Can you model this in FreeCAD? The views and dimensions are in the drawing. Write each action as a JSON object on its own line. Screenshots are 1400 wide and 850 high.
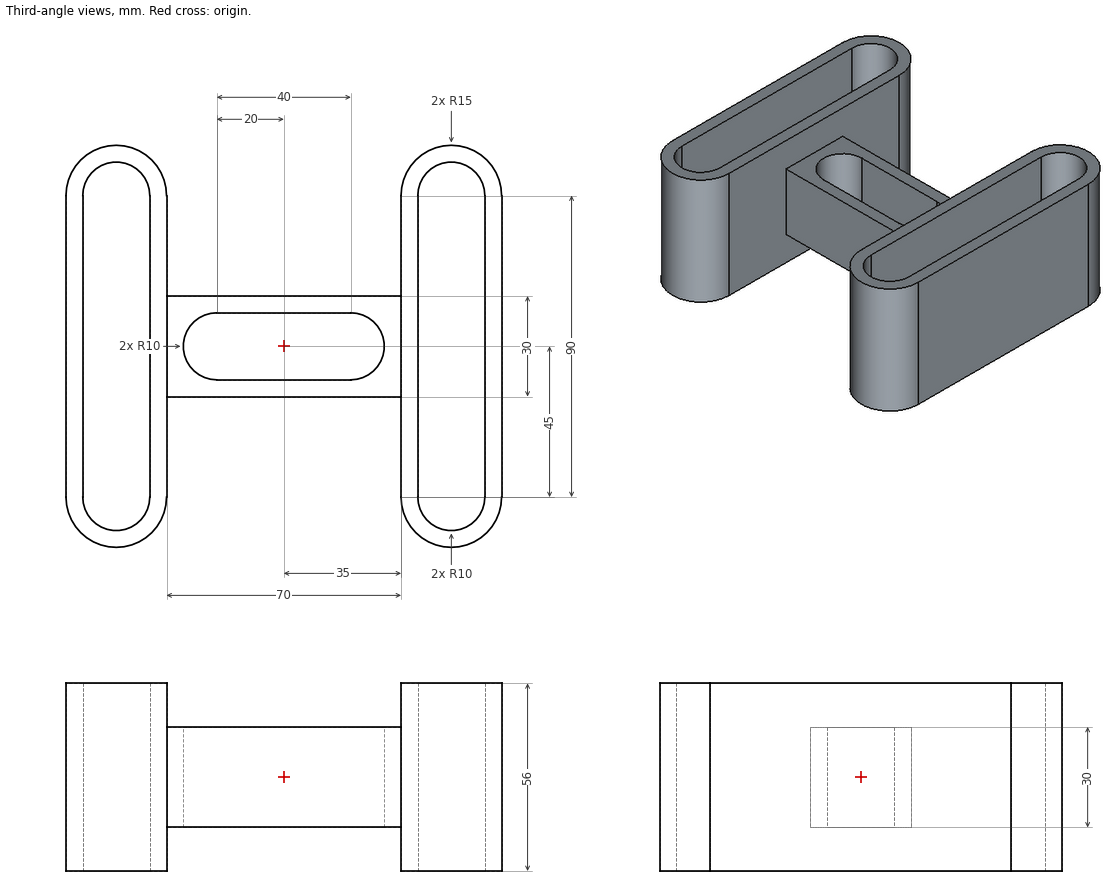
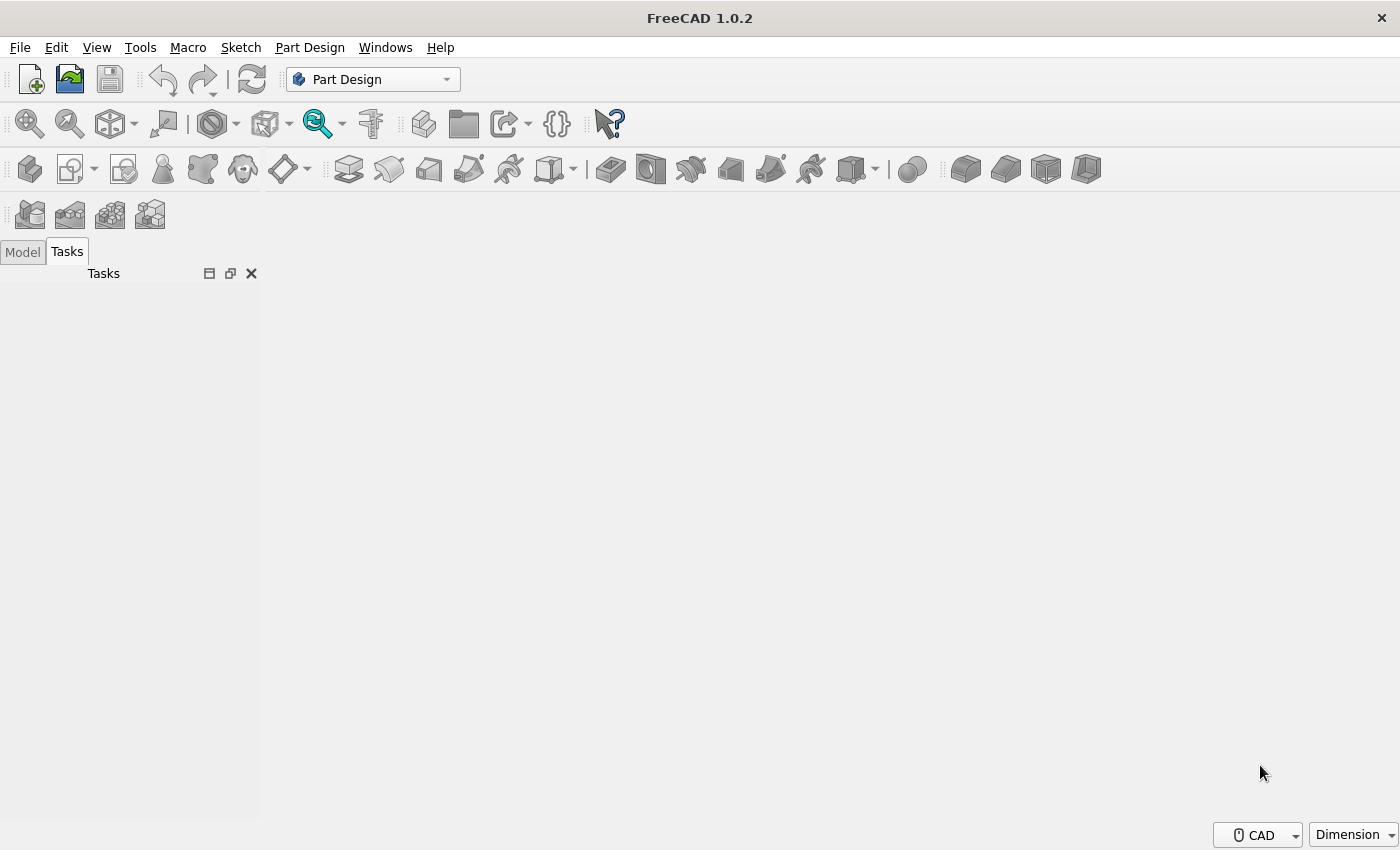
{"action": "left_click", "coordinate": [30, 80]}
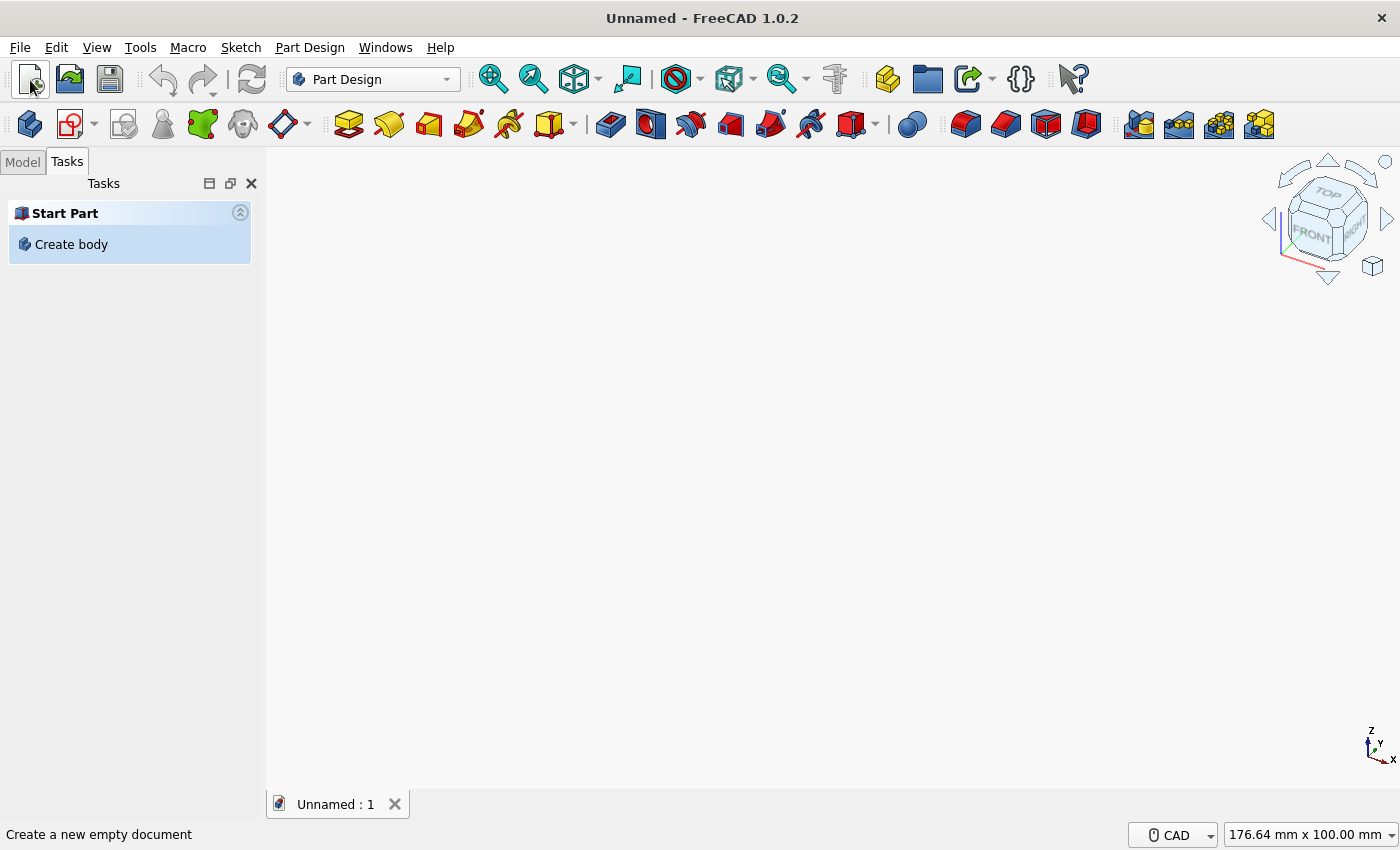
{"action": "left_click", "coordinate": [70, 124]}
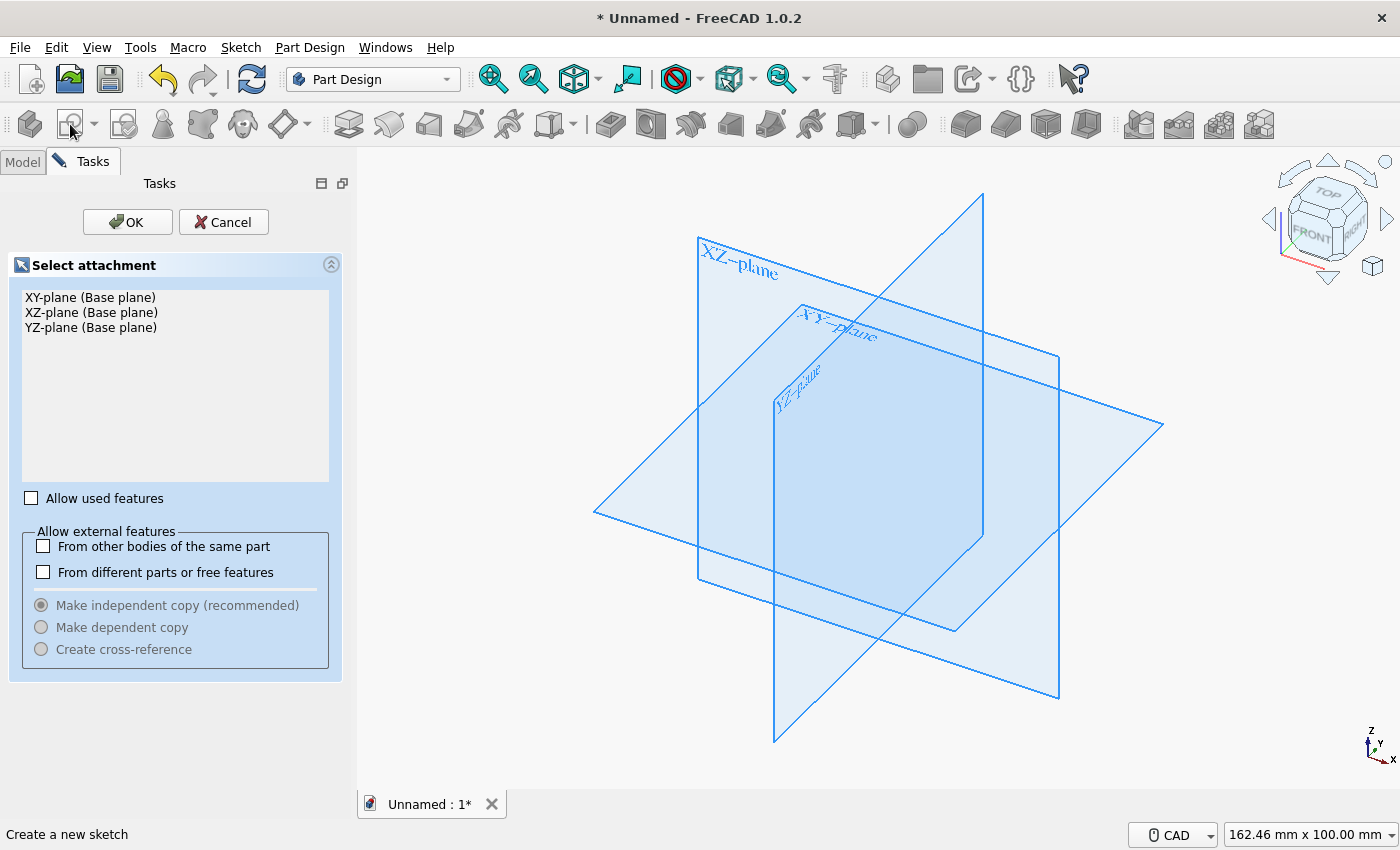
{"action": "left_click", "coordinate": [82, 298]}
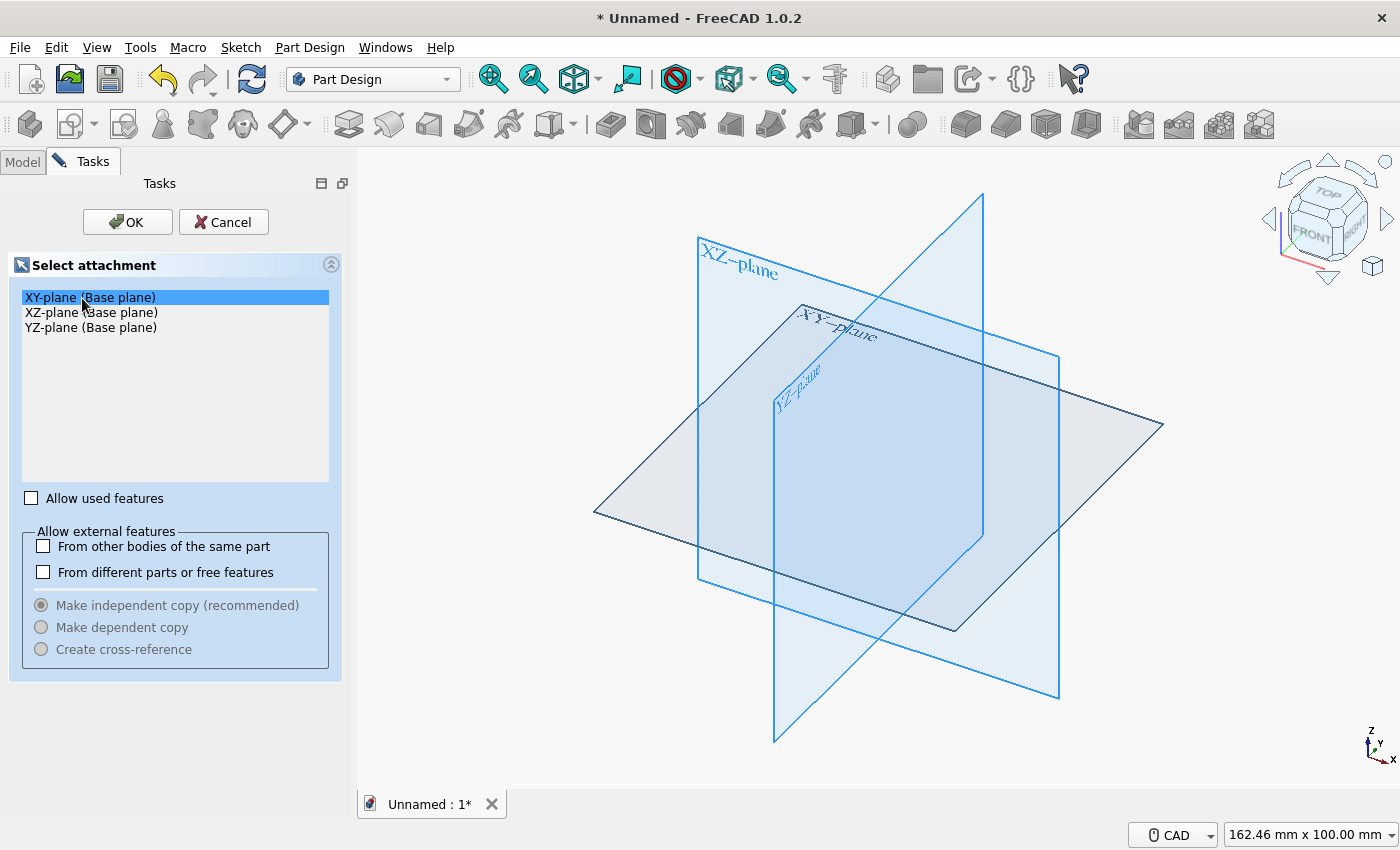
{"action": "left_click", "coordinate": [128, 222]}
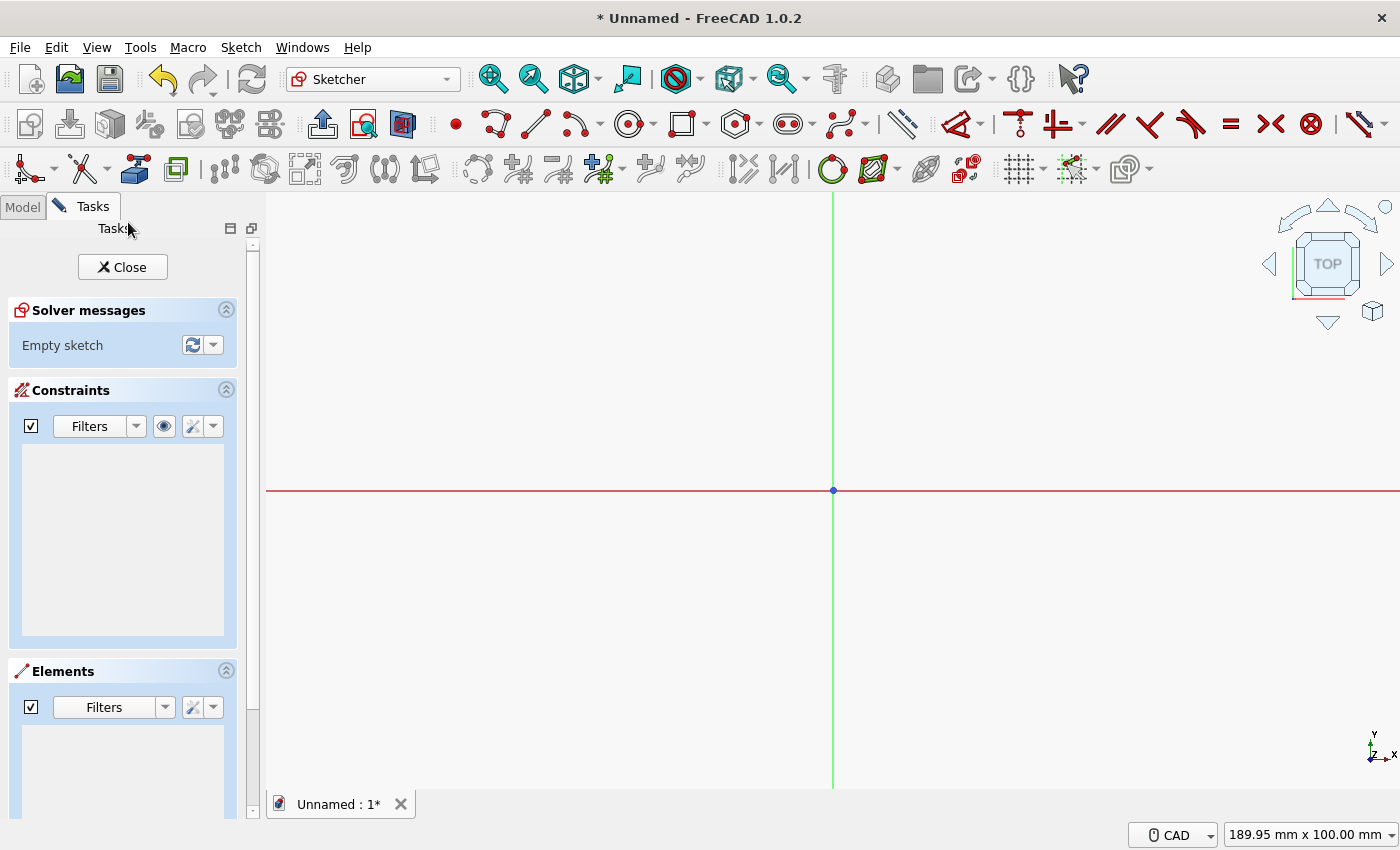
{"action": "scroll", "coordinate": [972, 490], "scroll_direction": "up", "scroll_amount": 2}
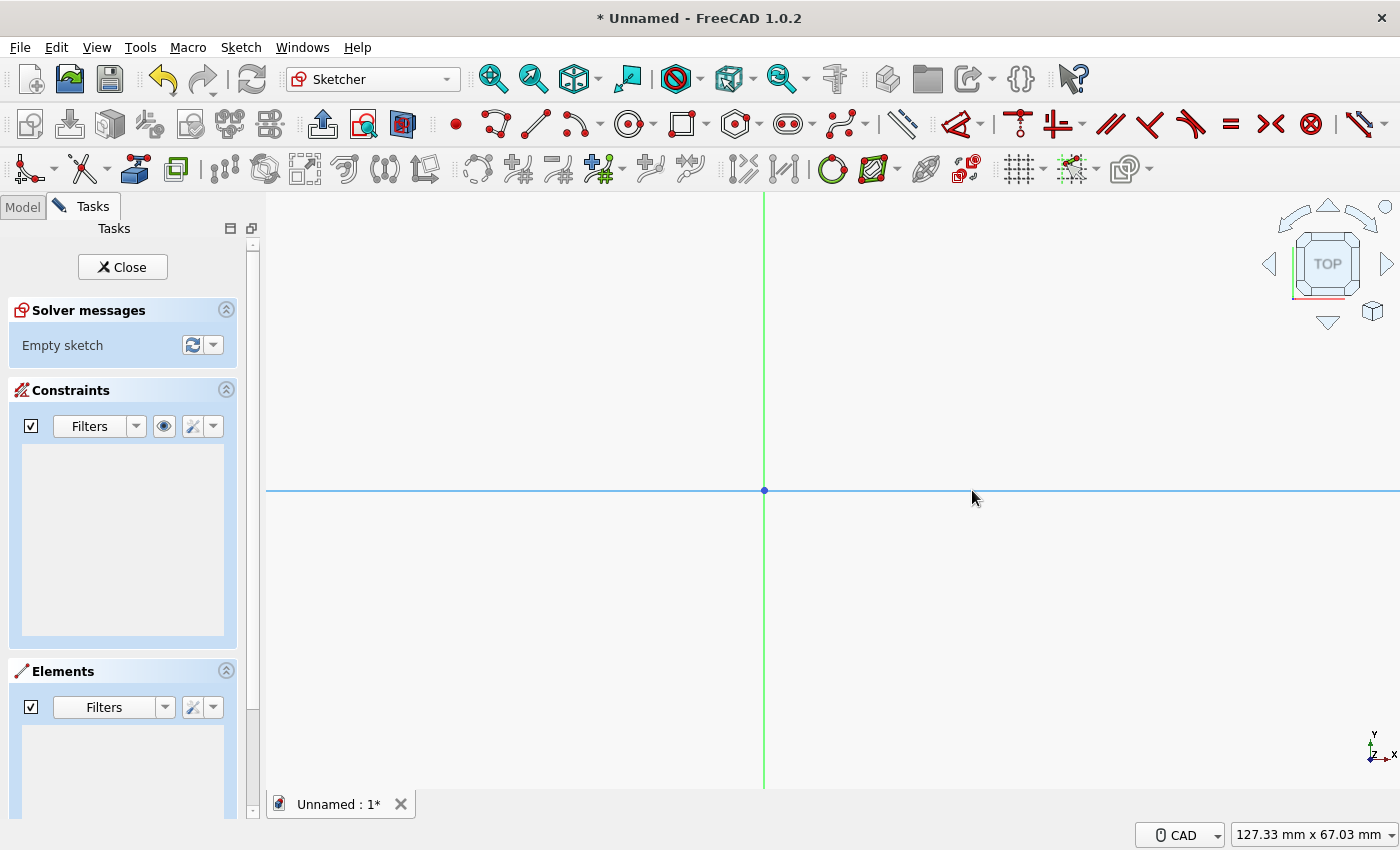
{"action": "key", "text": "g v"}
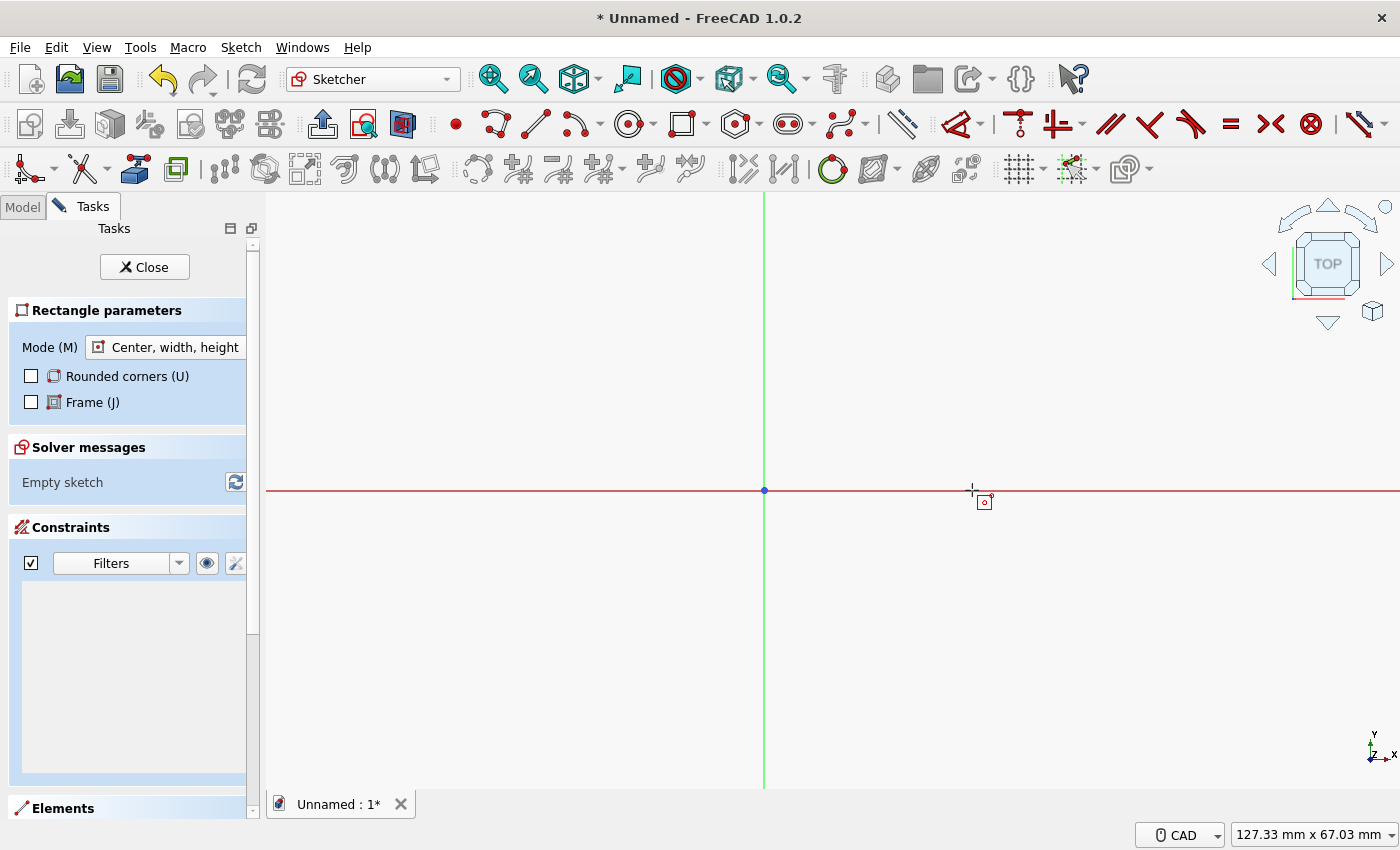
{"action": "left_click", "coordinate": [764, 490]}
{"action": "mouse_move", "coordinate": [1076, 357]}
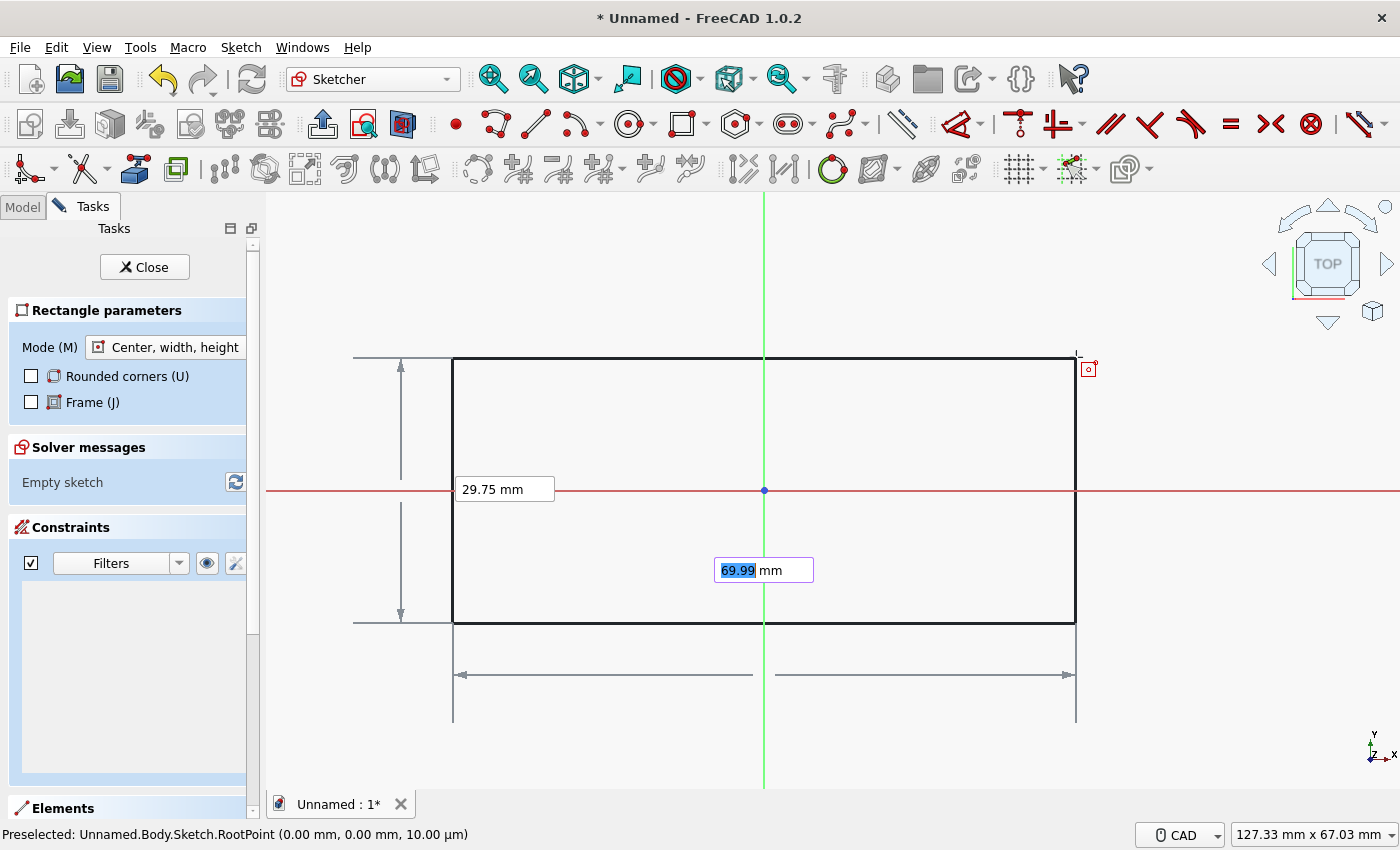
{"action": "type", "text": "70"}
{"action": "key", "text": "Tab"}
{"action": "type", "text": "30"}
{"action": "key", "text": "Return"}
{"action": "key", "text": "Escape"}